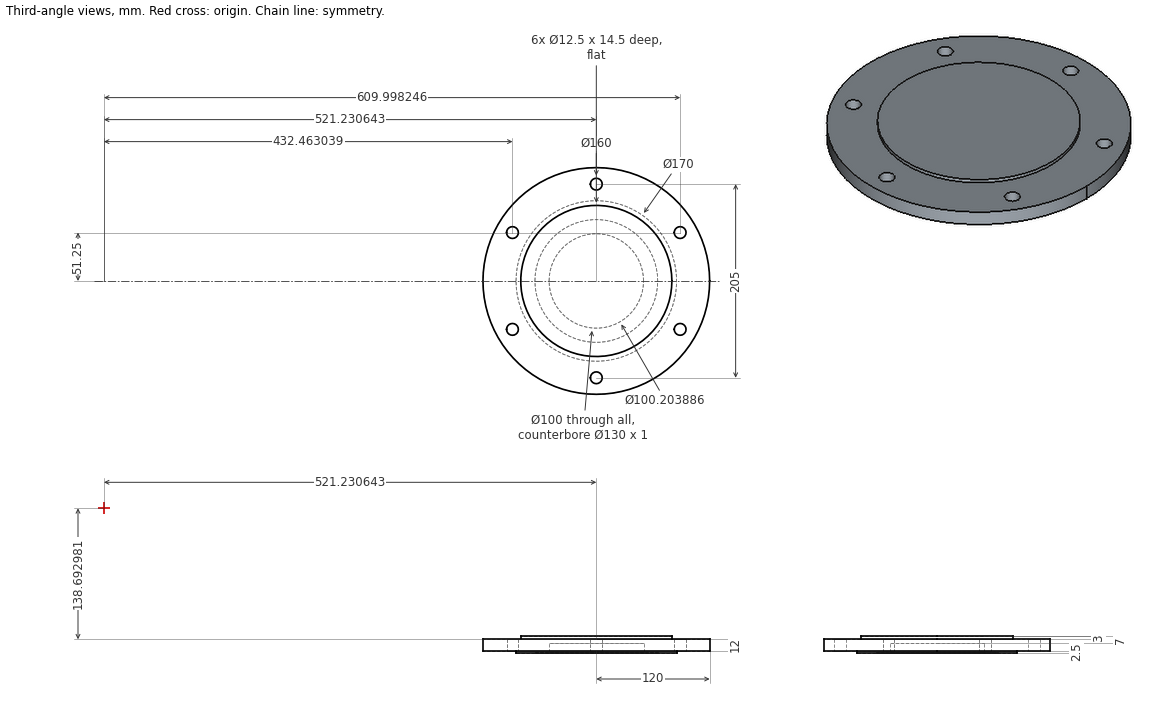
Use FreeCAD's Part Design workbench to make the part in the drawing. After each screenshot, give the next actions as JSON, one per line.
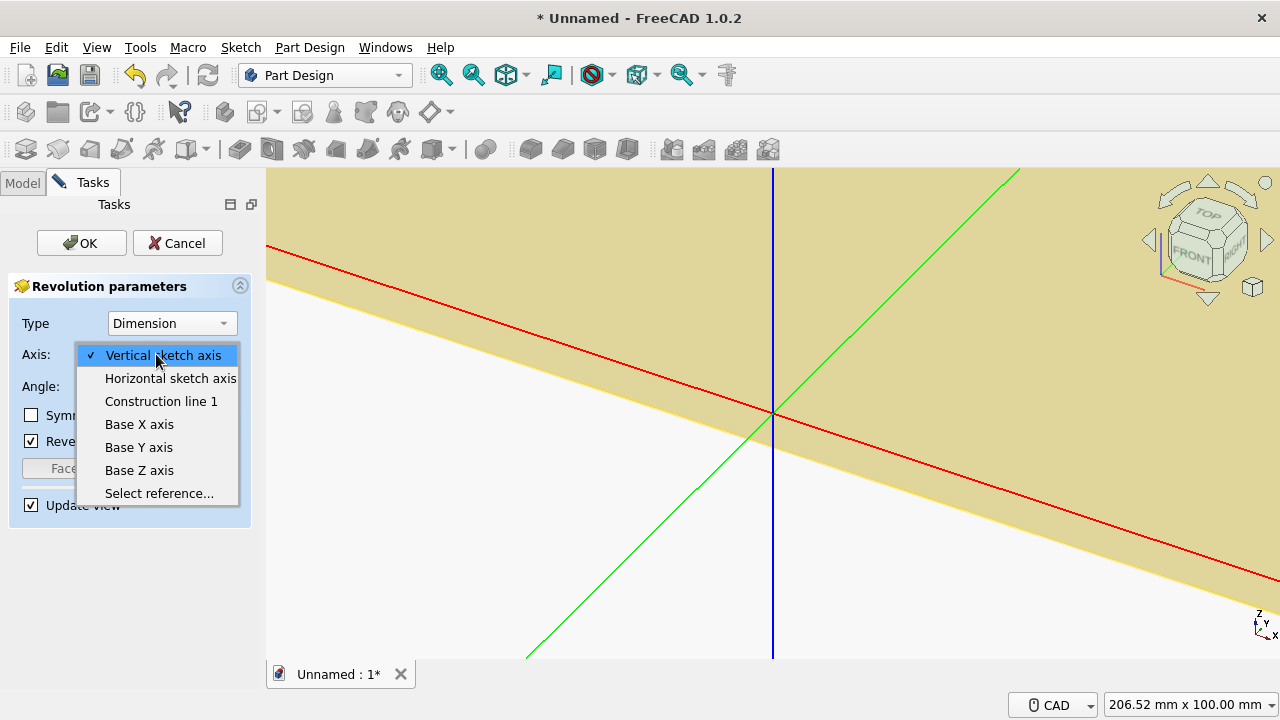
{"action": "left_click", "coordinate": [156, 402]}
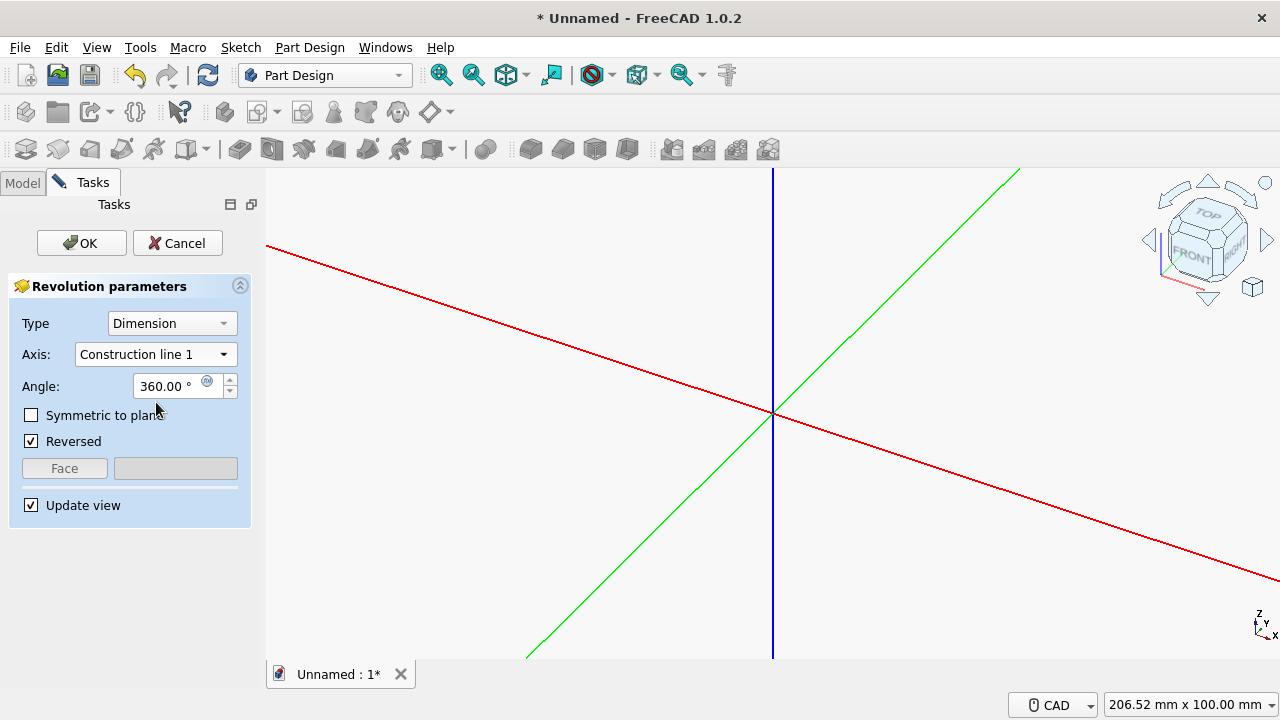
{"action": "left_click", "coordinate": [82, 243]}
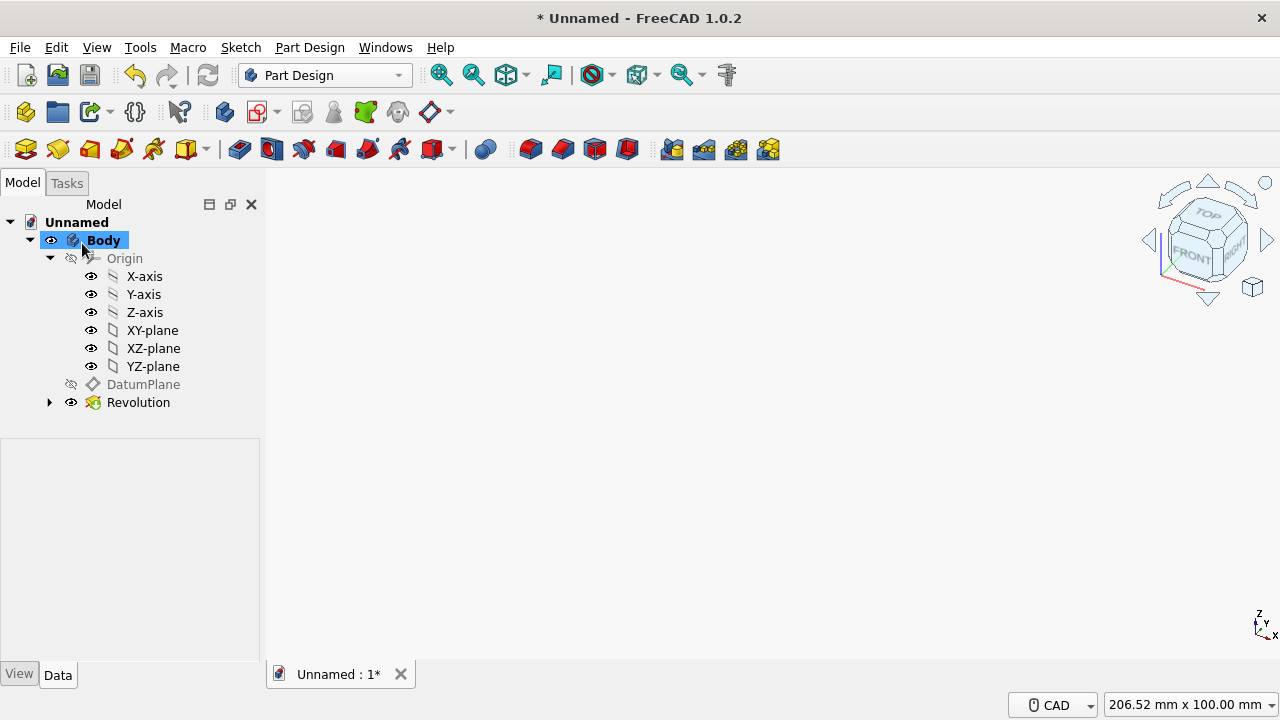
{"action": "key", "text": "v f"}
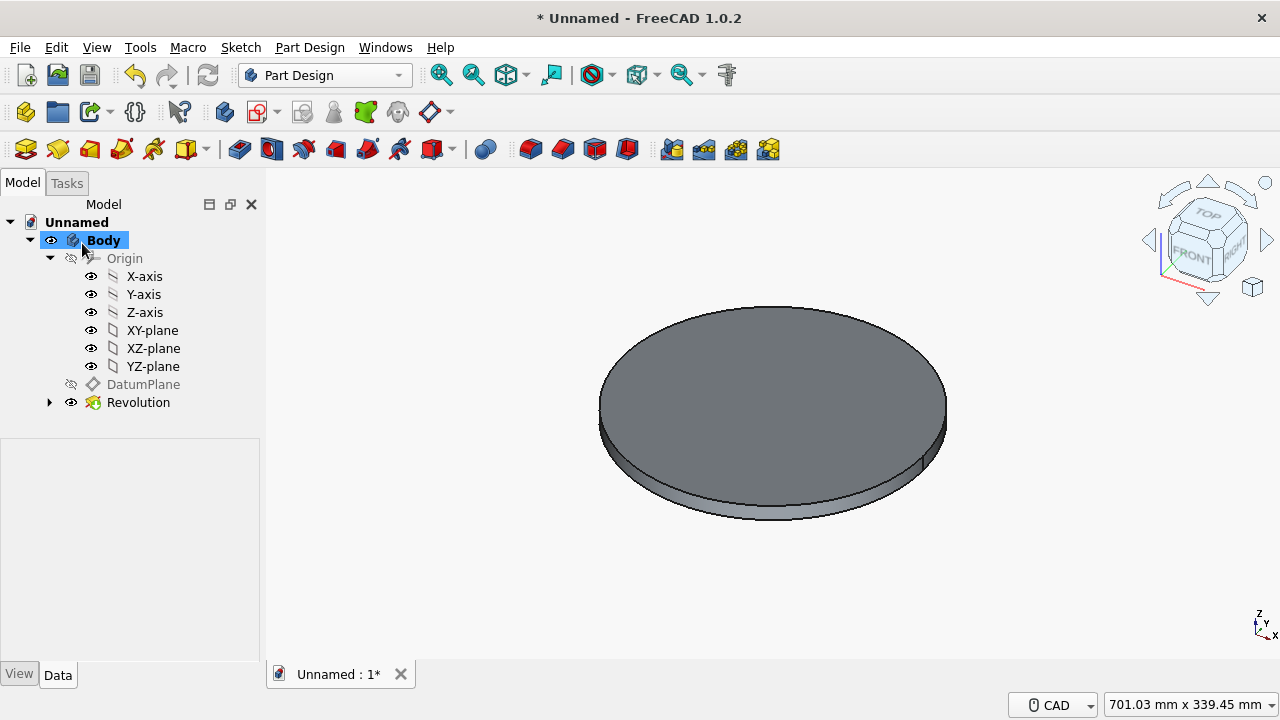
{"action": "key", "text": "5"}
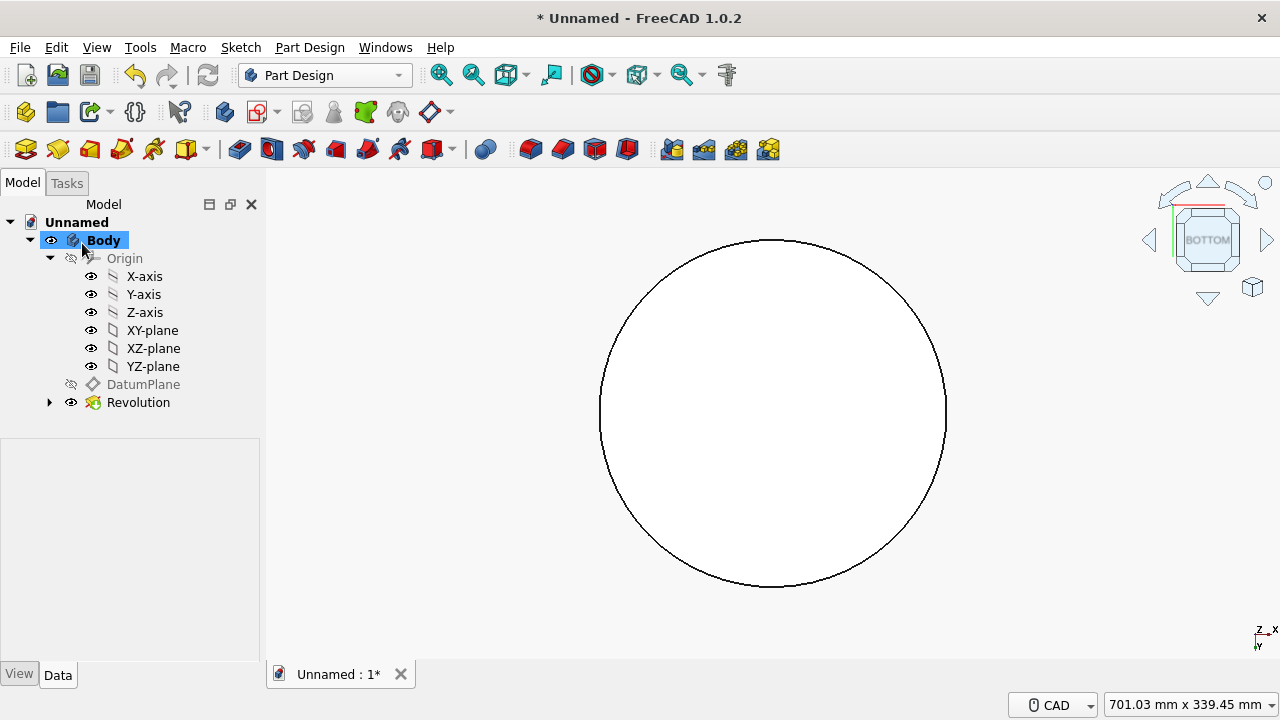
{"action": "left_click", "coordinate": [773, 412]}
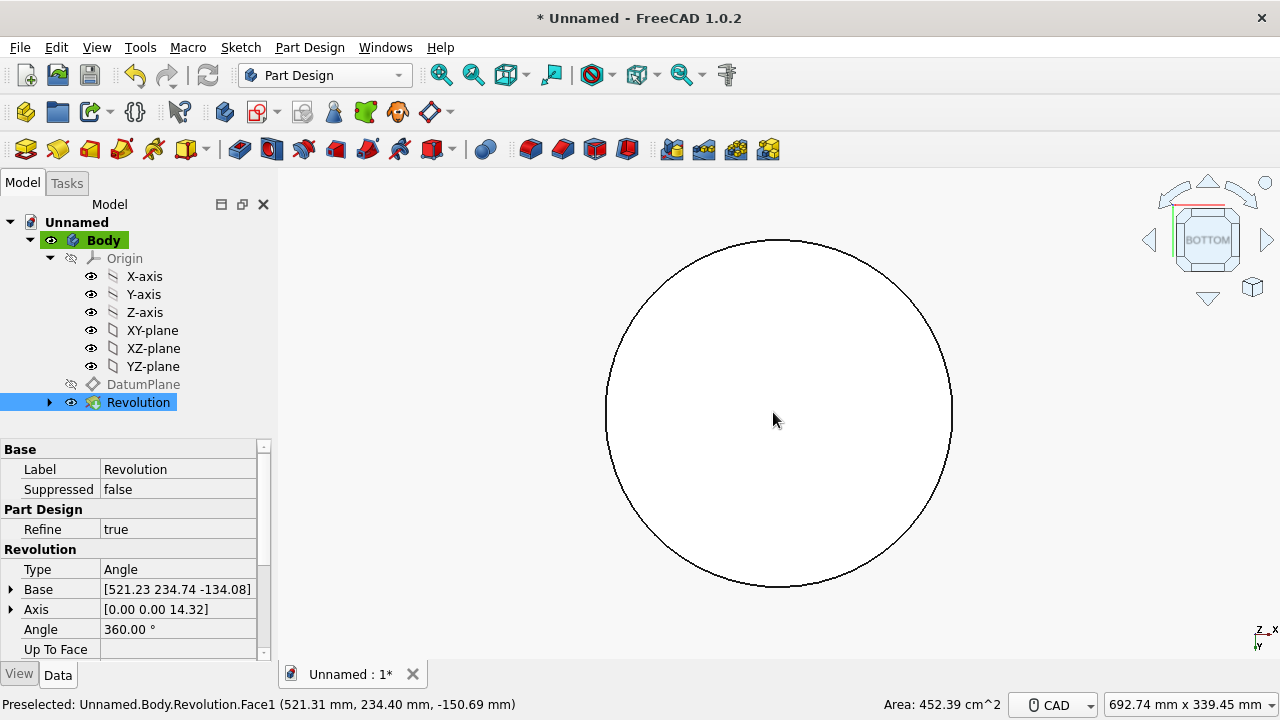
{"action": "left_click", "coordinate": [258, 112]}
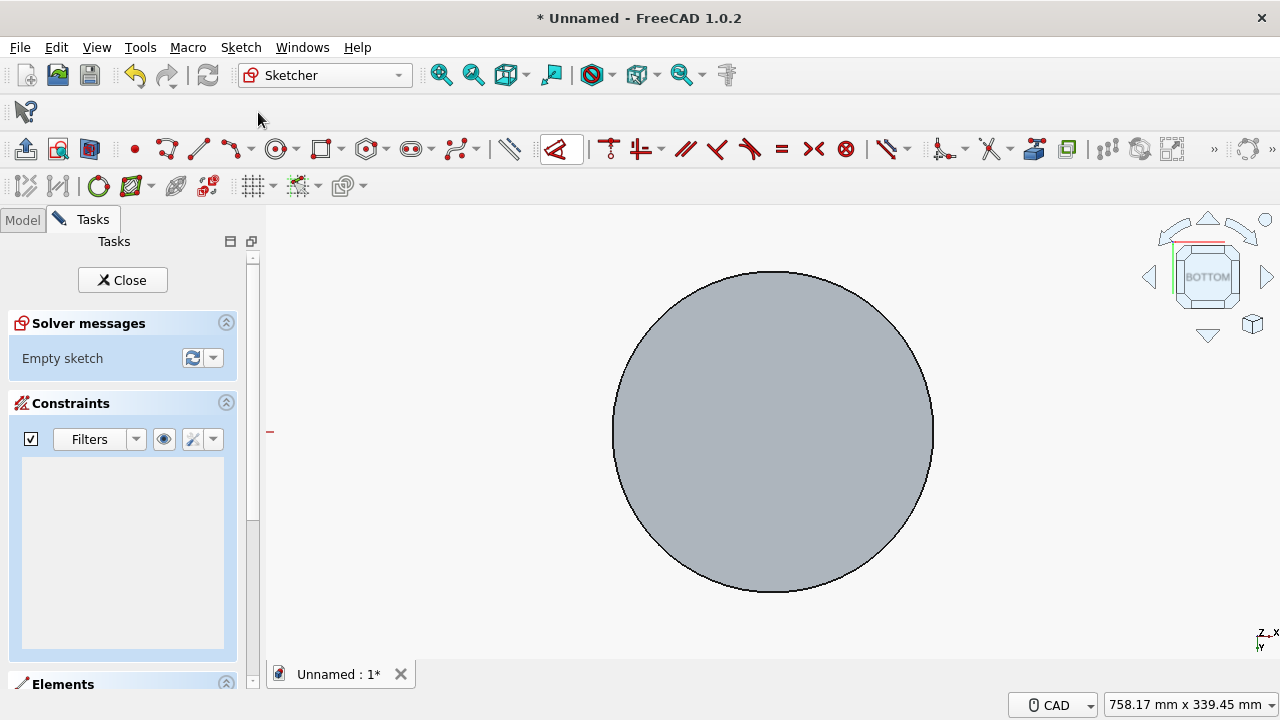
{"action": "key", "text": "g c"}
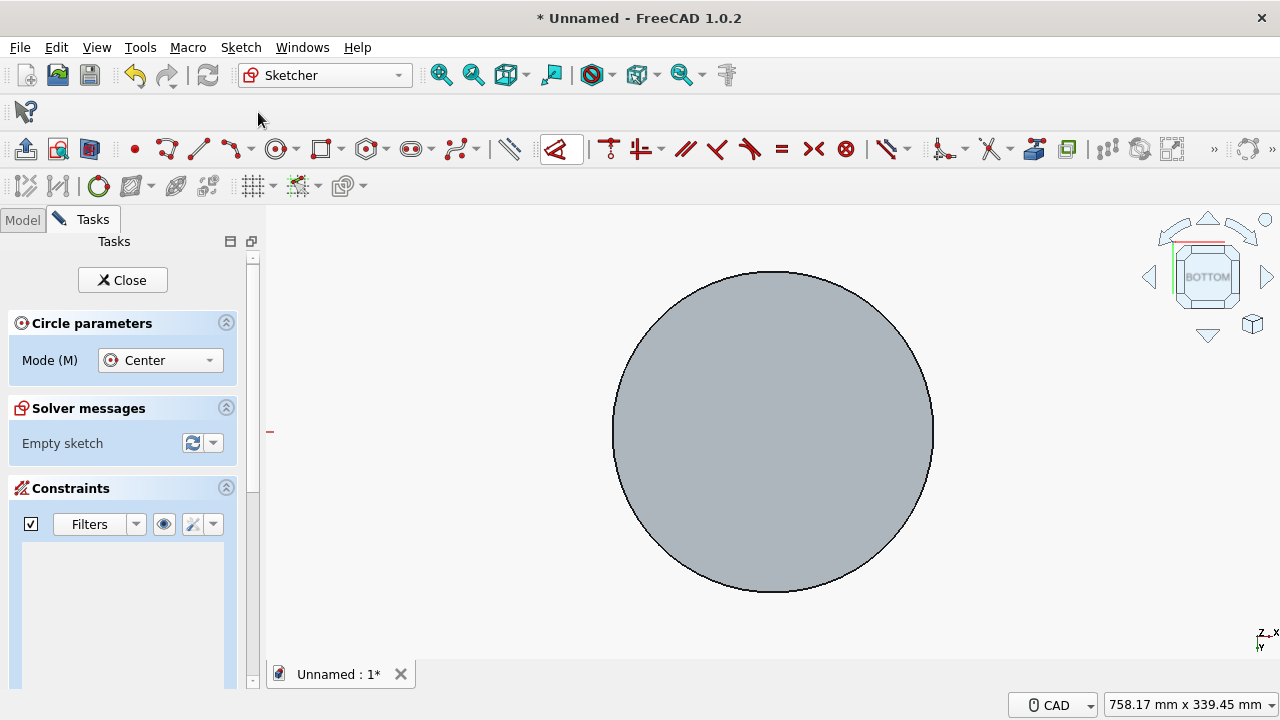
{"action": "left_click", "coordinate": [773, 432]}
{"action": "mouse_move", "coordinate": [853, 352]}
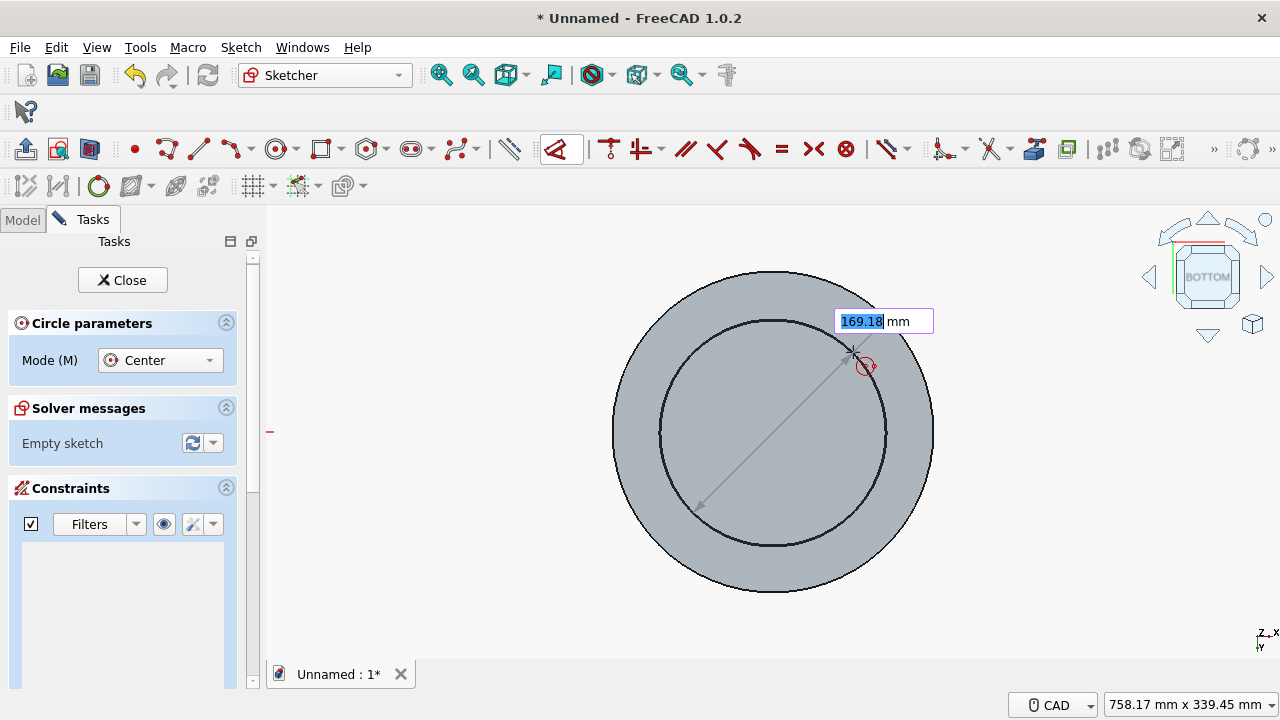
{"action": "type", "text": "170"}
{"action": "key", "text": "Return"}
{"action": "key", "text": "Escape"}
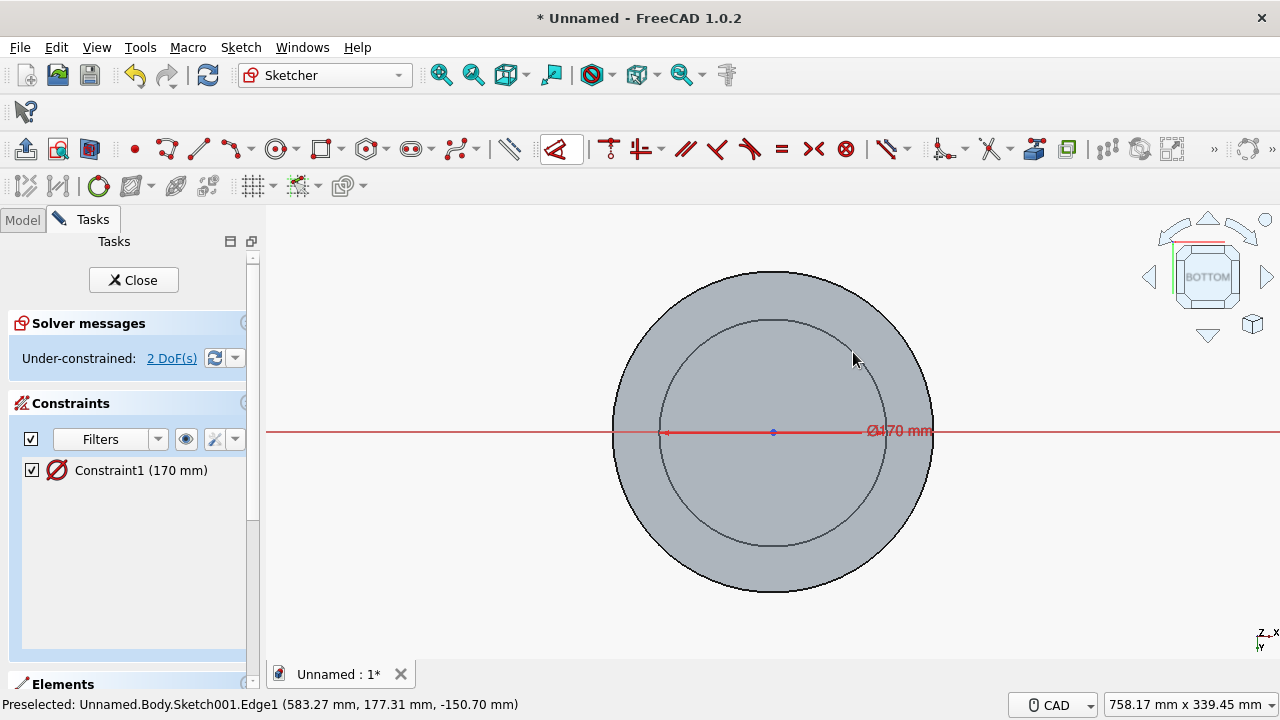
{"action": "left_click", "coordinate": [773, 433]}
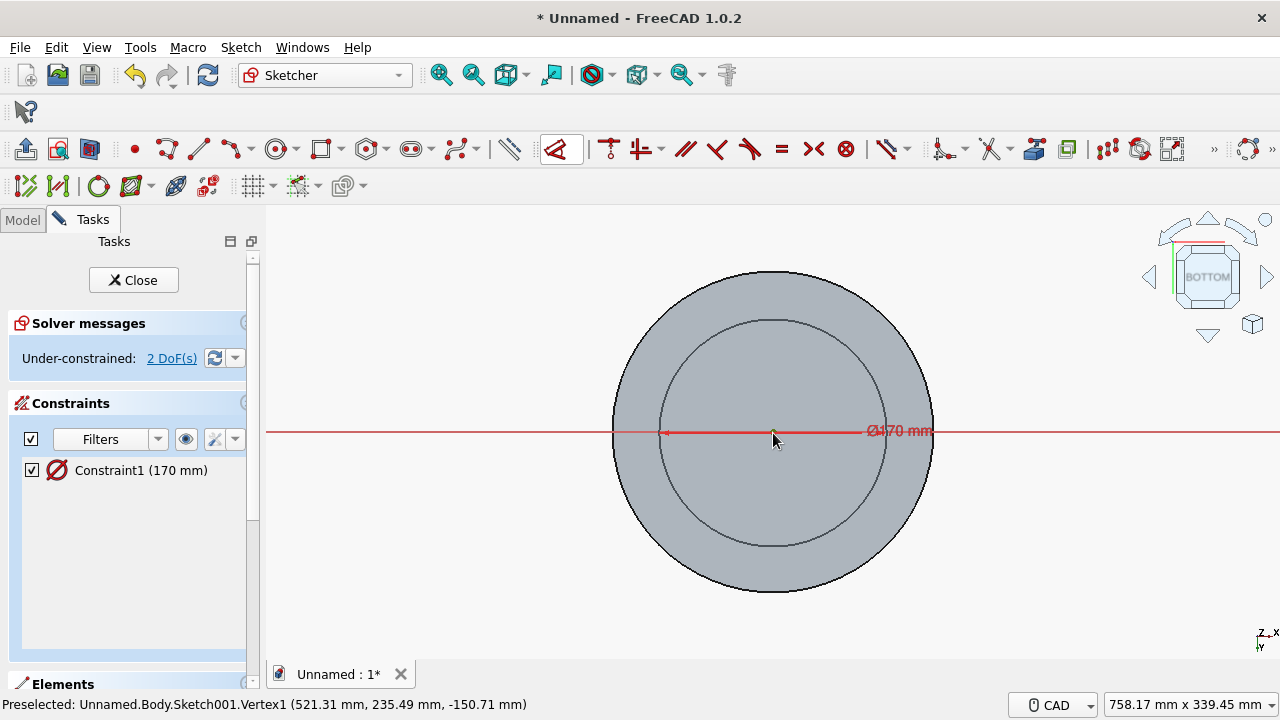
{"action": "left_click", "coordinate": [353, 432]}